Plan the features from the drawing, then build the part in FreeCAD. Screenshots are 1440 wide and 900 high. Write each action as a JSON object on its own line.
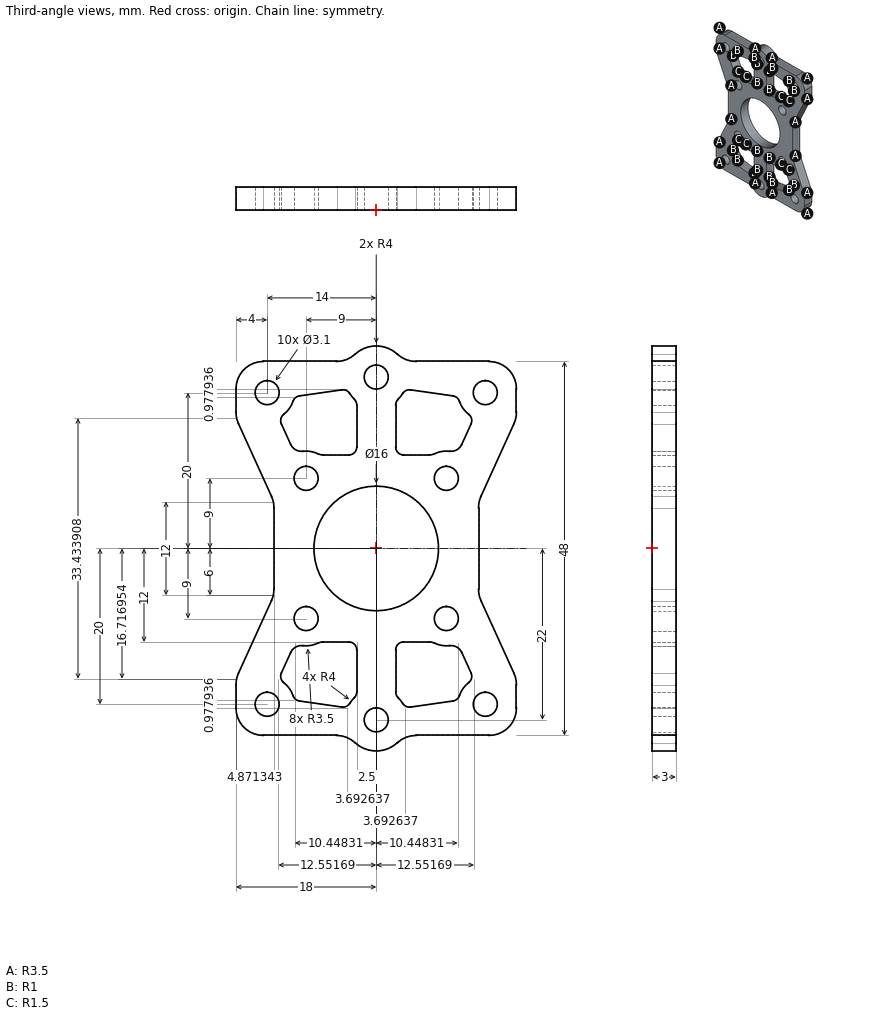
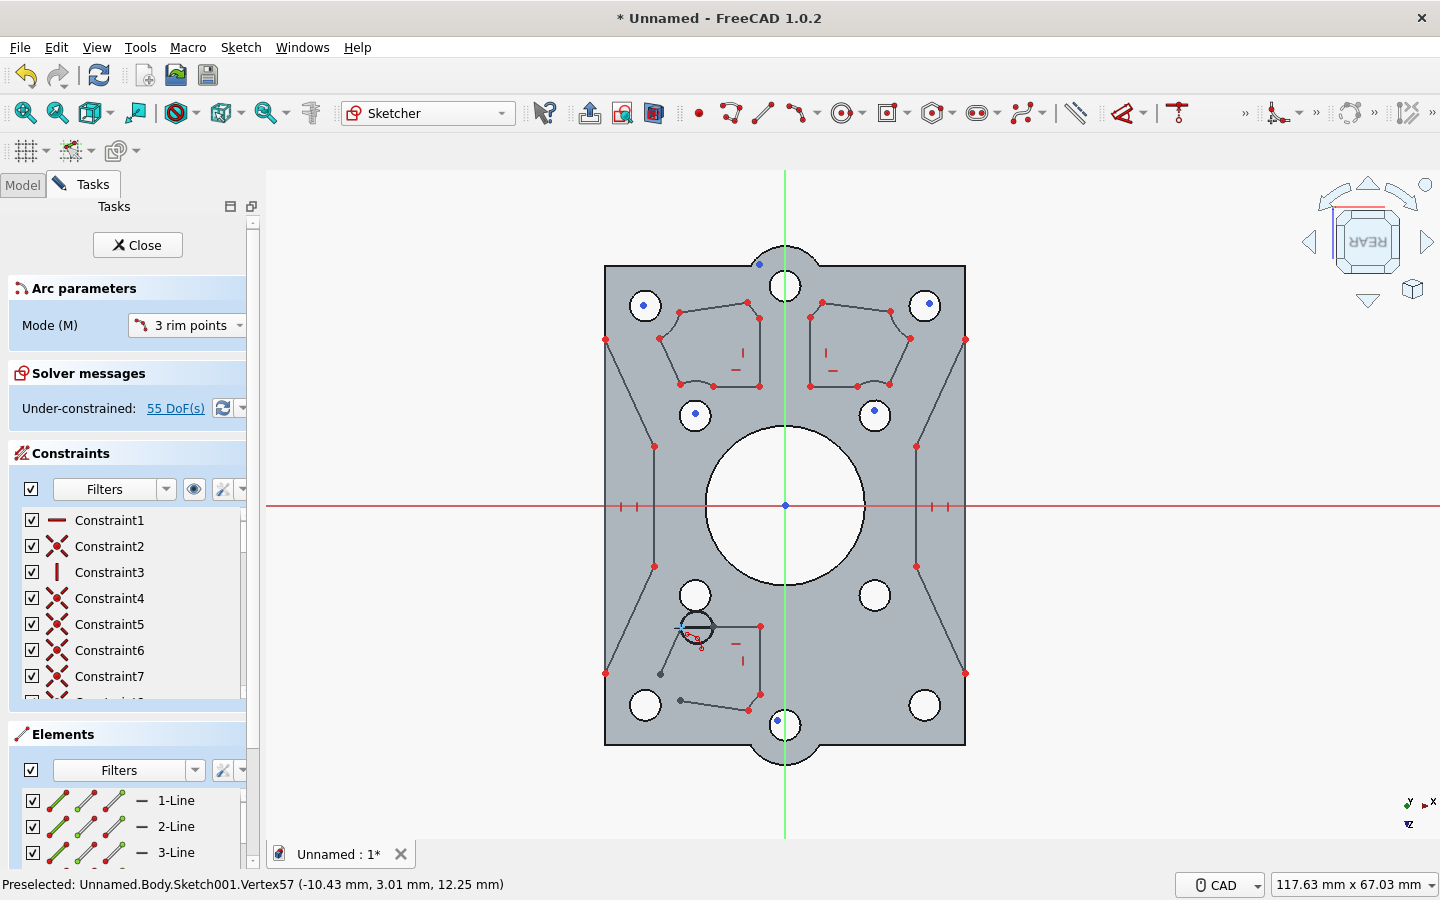
{"action": "scroll", "coordinate": [697, 630], "scroll_direction": "up", "scroll_amount": 7}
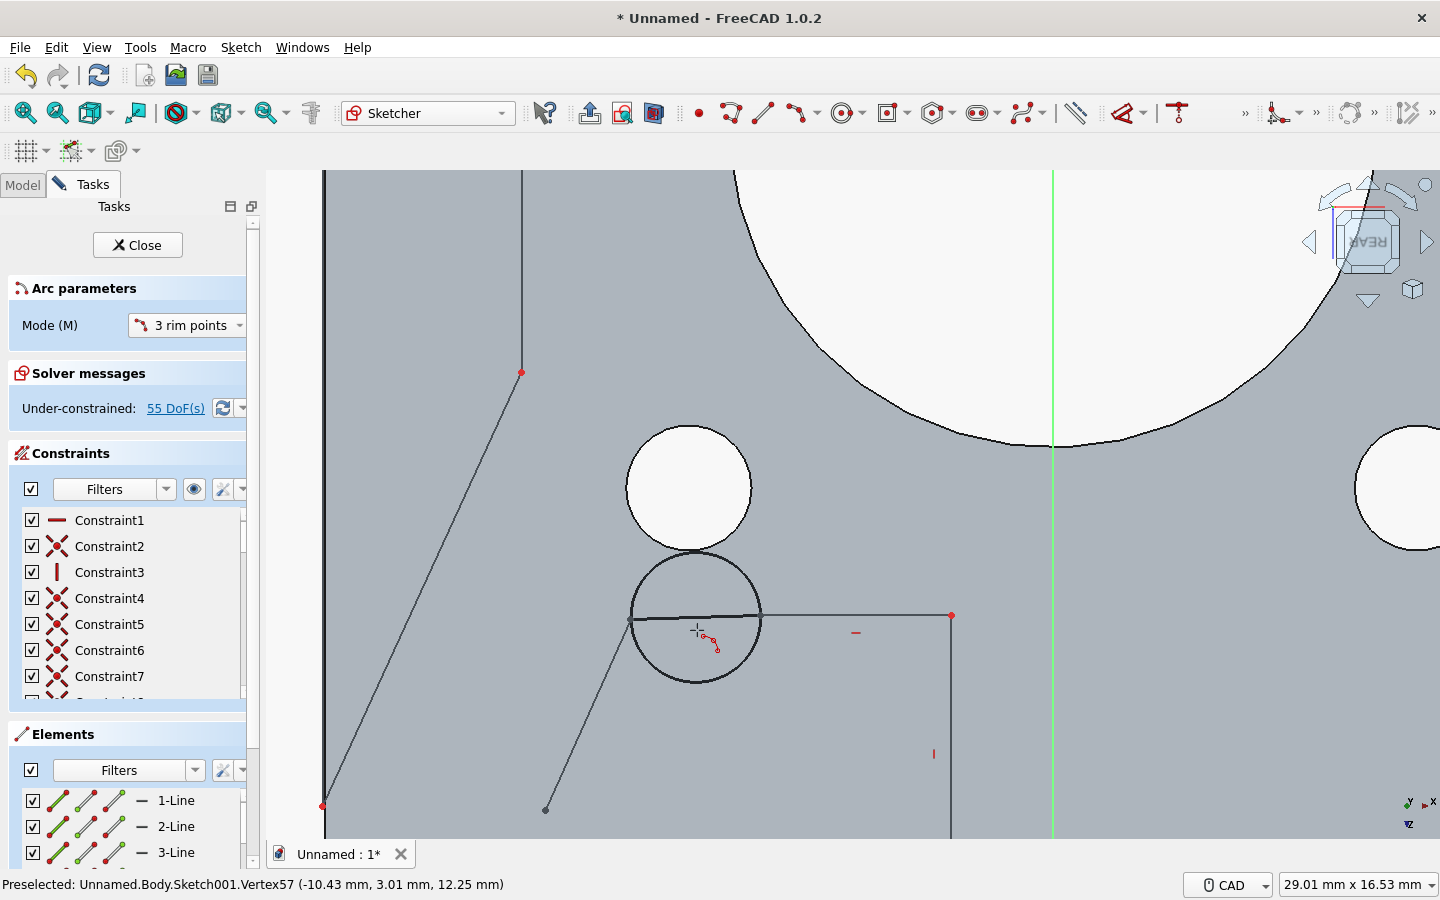
{"action": "left_click", "coordinate": [697, 629]}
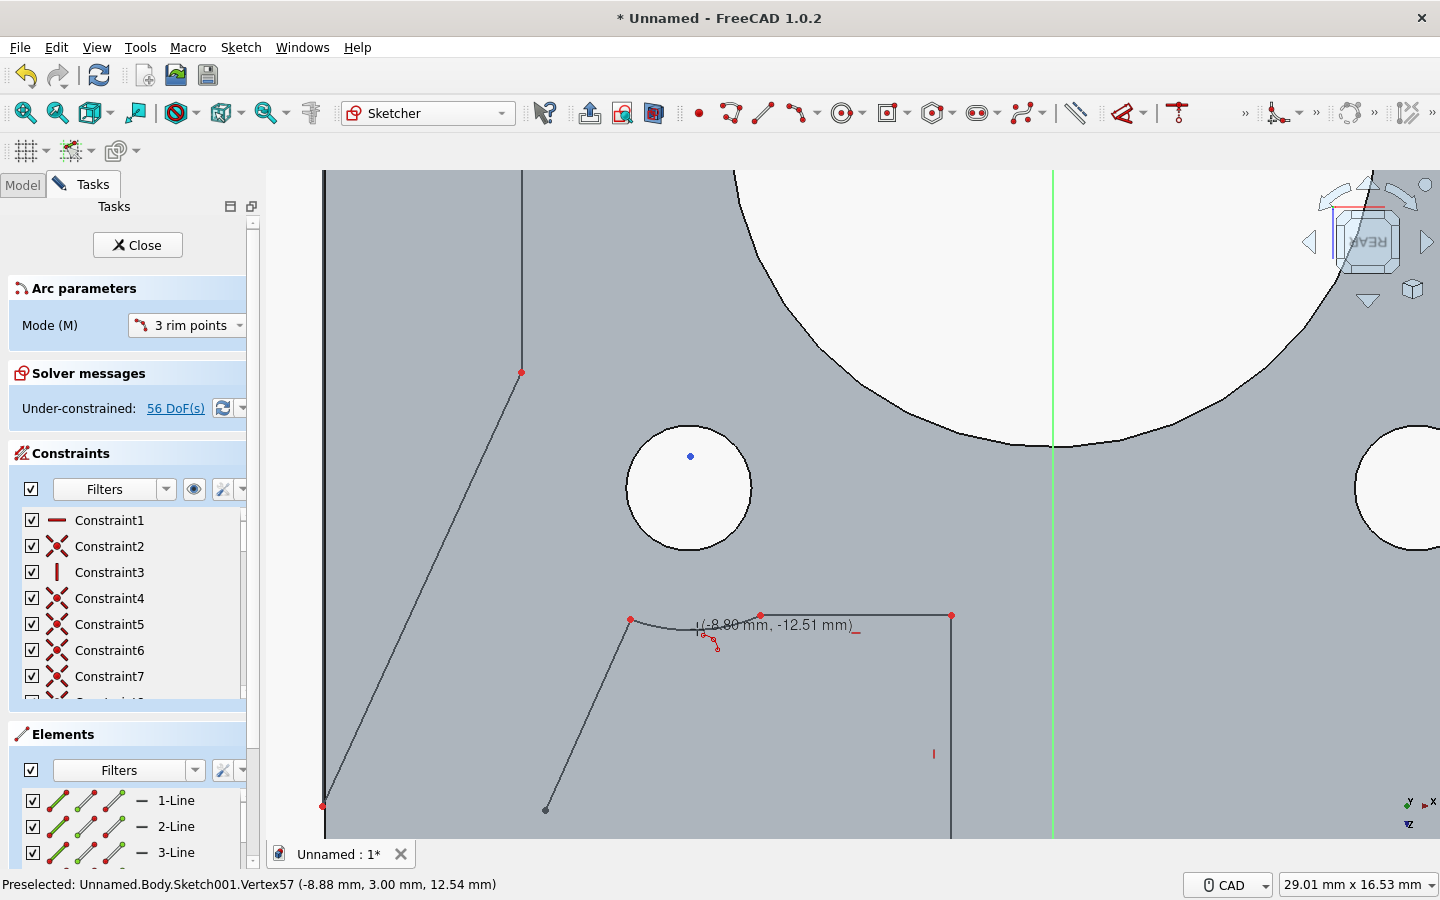
{"action": "scroll", "coordinate": [697, 629], "scroll_direction": "down", "scroll_amount": 7}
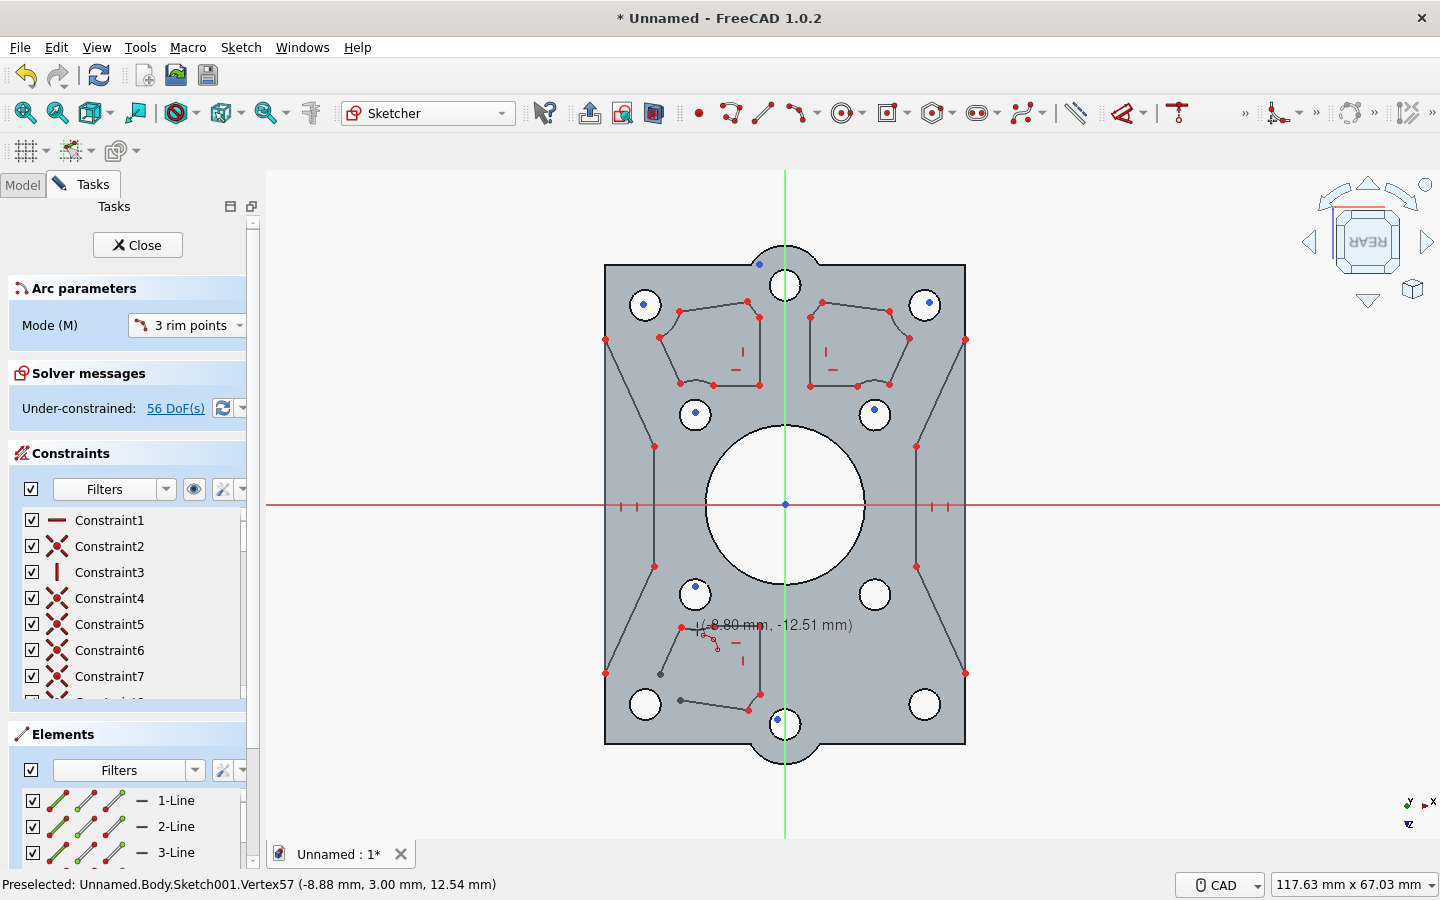
{"action": "left_click", "coordinate": [660, 674]}
{"action": "left_click", "coordinate": [680, 700]}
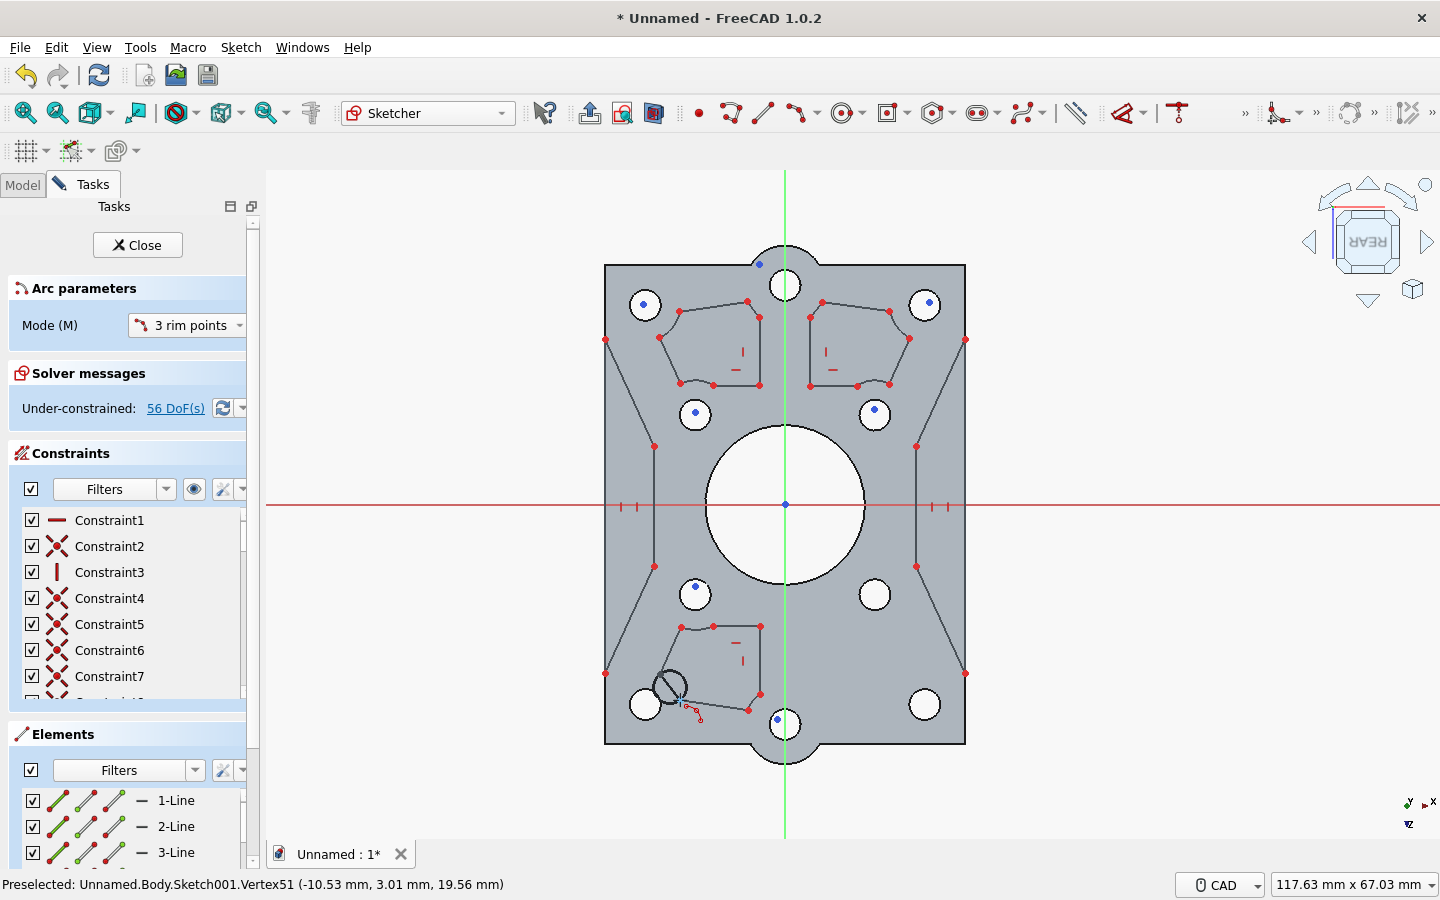
{"action": "scroll", "coordinate": [673, 684], "scroll_direction": "up", "scroll_amount": 7}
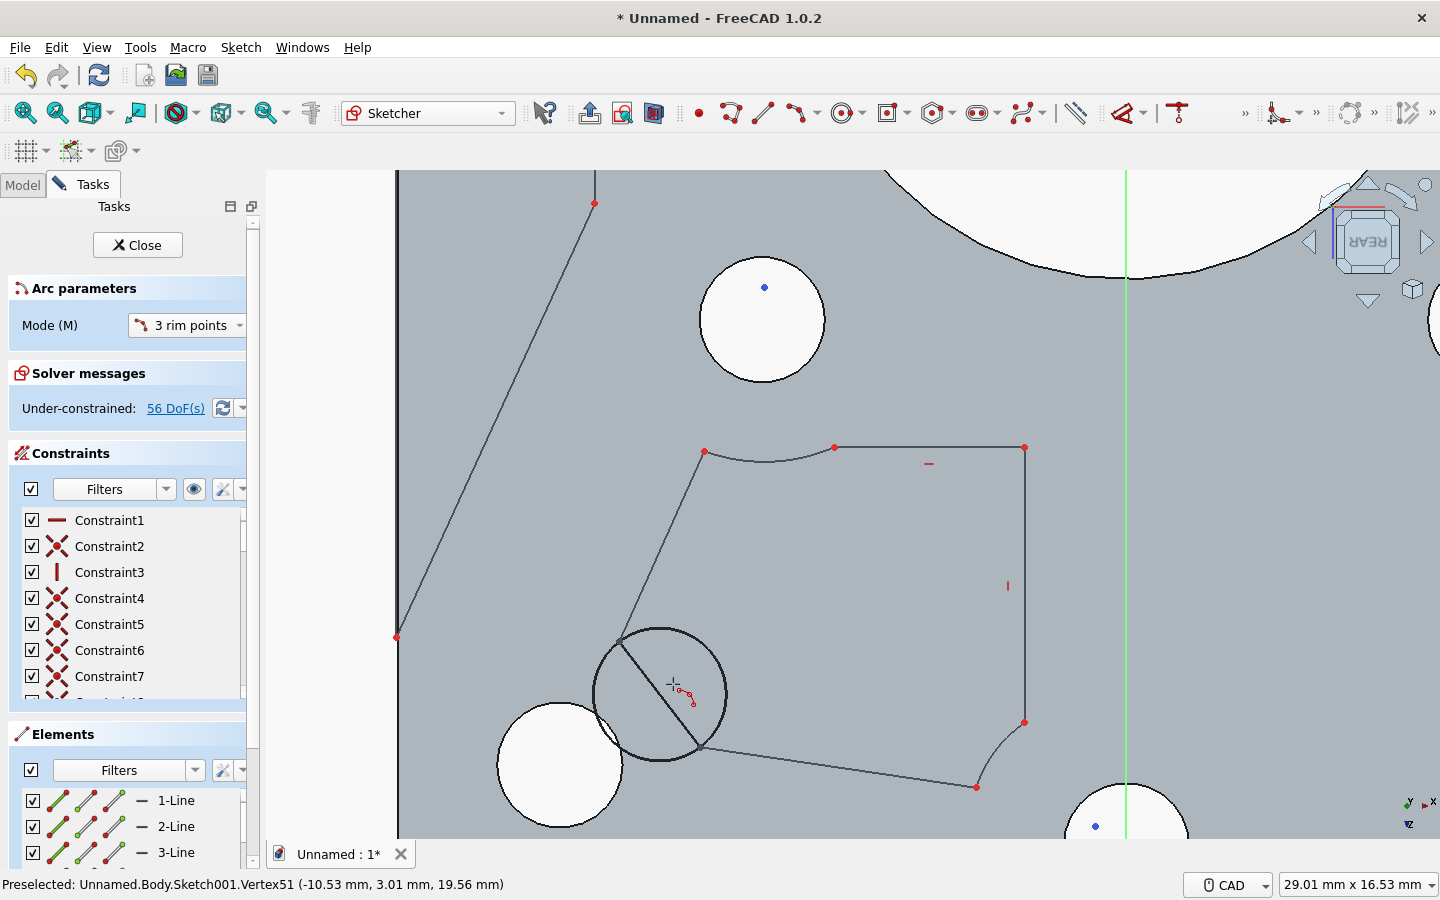
{"action": "left_click", "coordinate": [673, 680]}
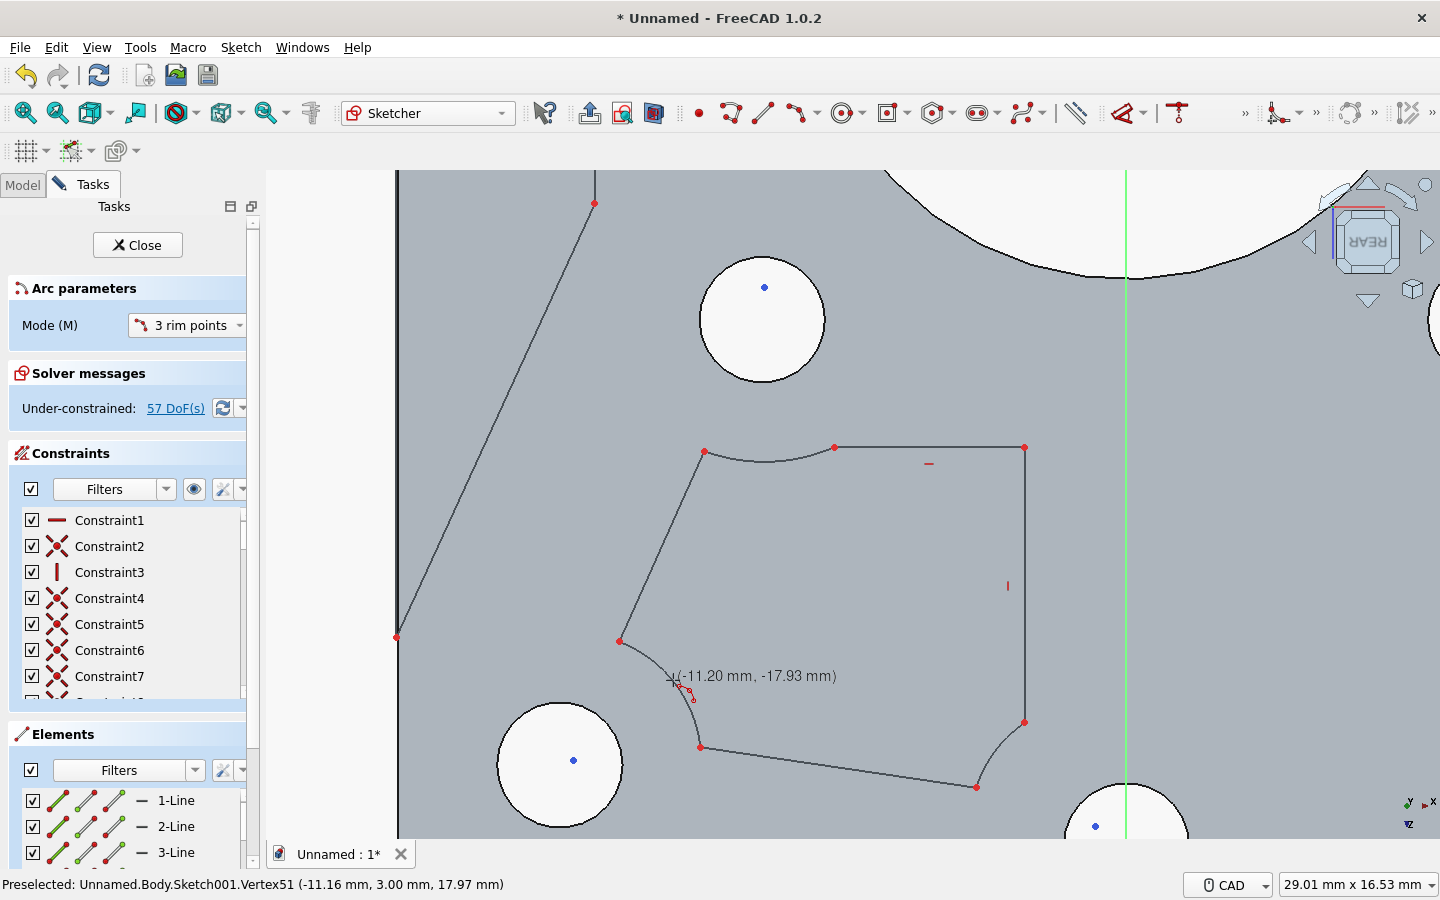
{"action": "left_click", "coordinate": [764, 114]}